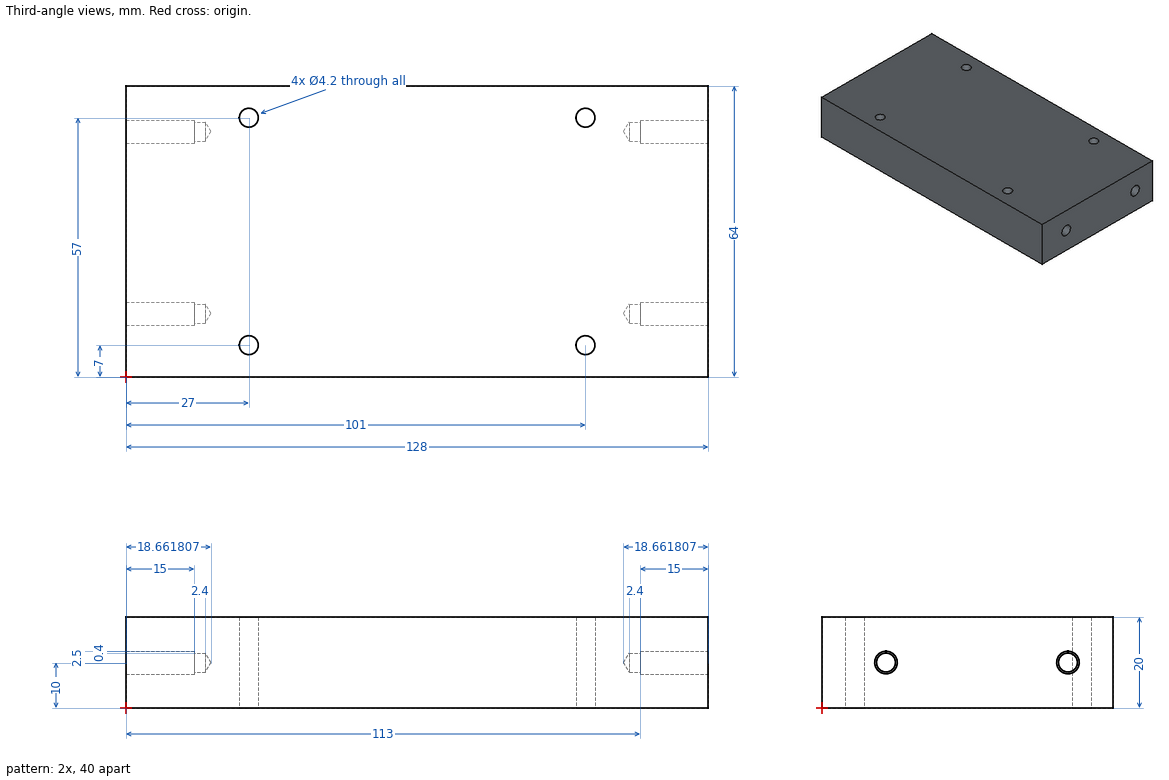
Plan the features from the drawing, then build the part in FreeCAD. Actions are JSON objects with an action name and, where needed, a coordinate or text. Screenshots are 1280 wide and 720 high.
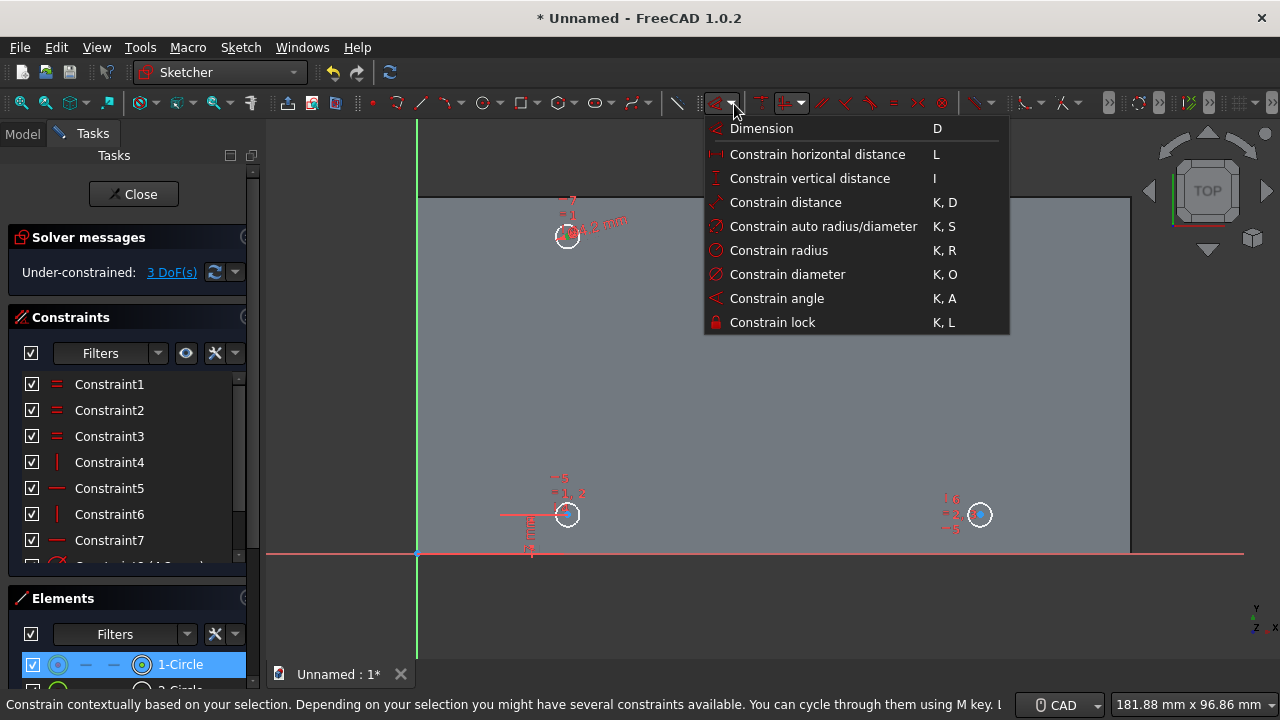
{"action": "left_click", "coordinate": [857, 154]}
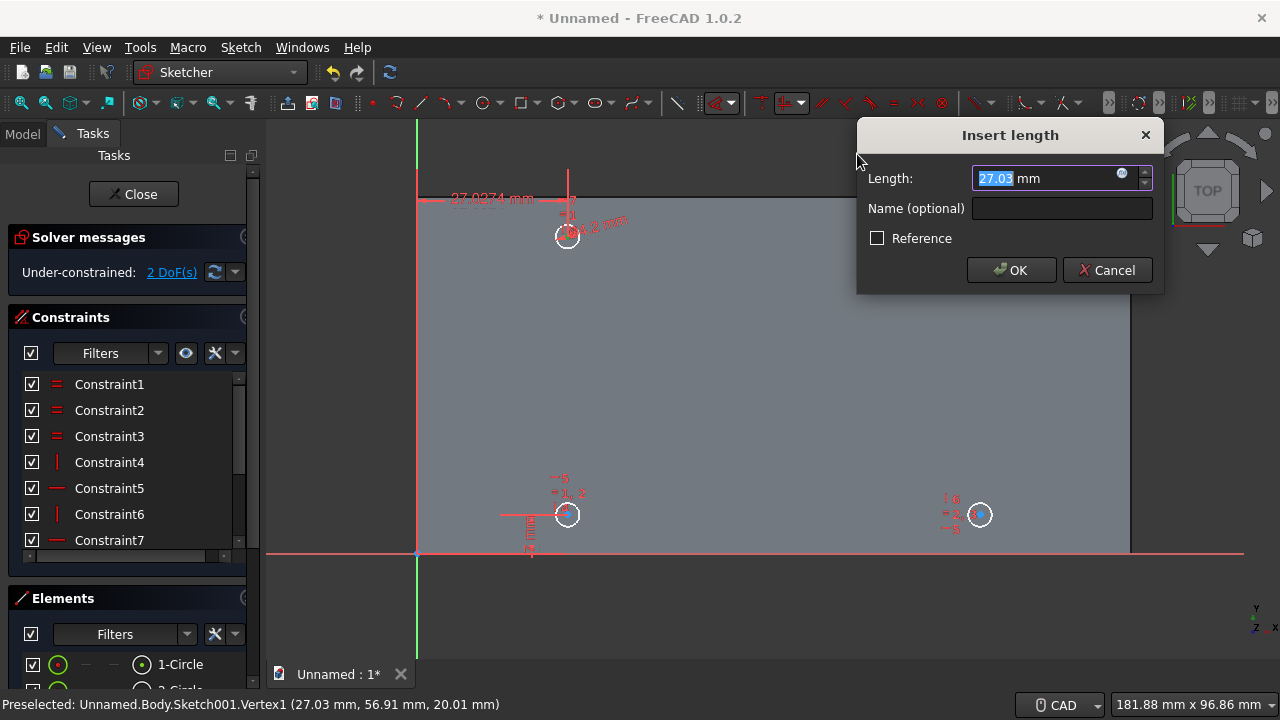
{"action": "type", "text": "27"}
{"action": "key", "text": "Return"}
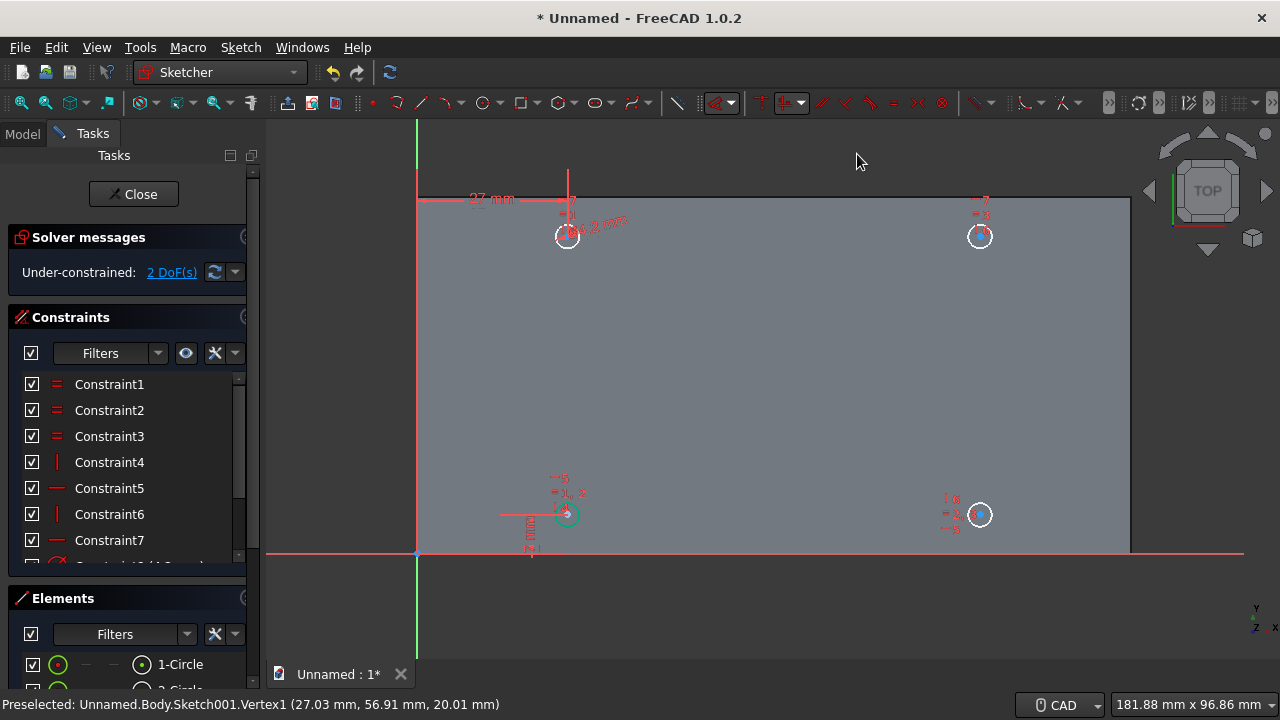
{"action": "left_click", "coordinate": [568, 237]}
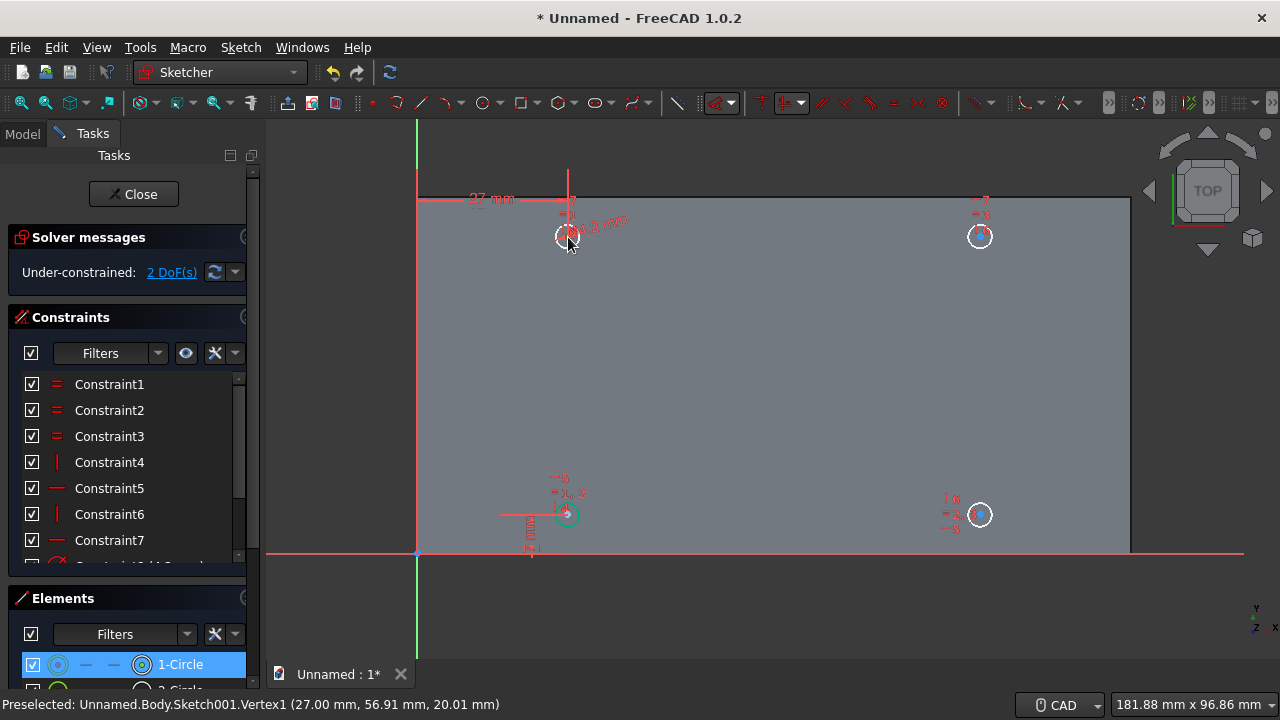
{"action": "left_click", "coordinate": [734, 104]}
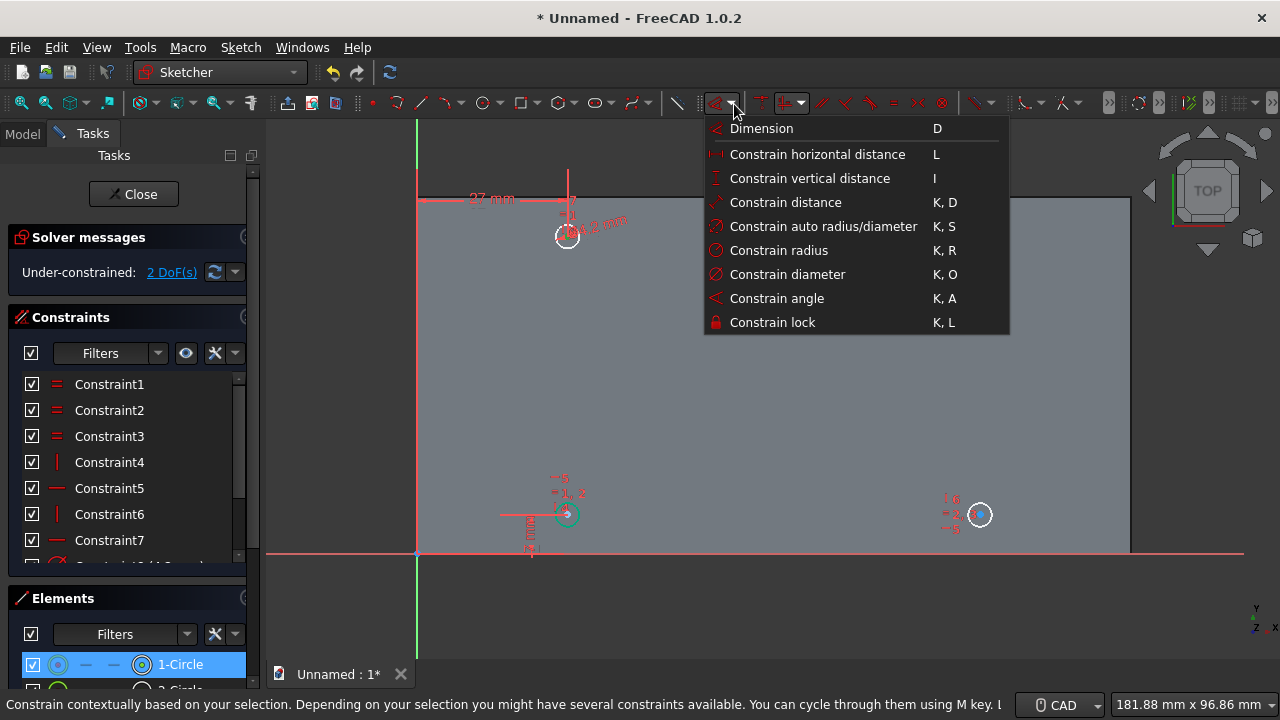
{"action": "left_click", "coordinate": [857, 178]}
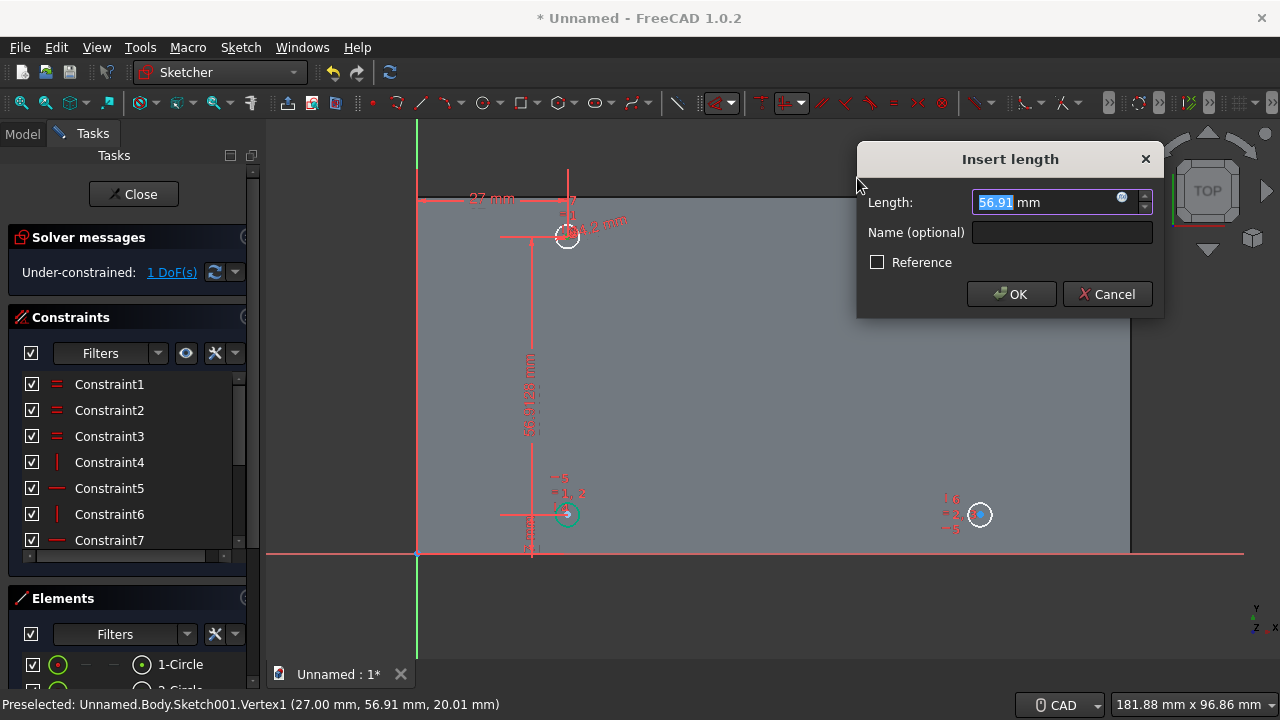
{"action": "type", "text": "57"}
{"action": "key", "text": "Return"}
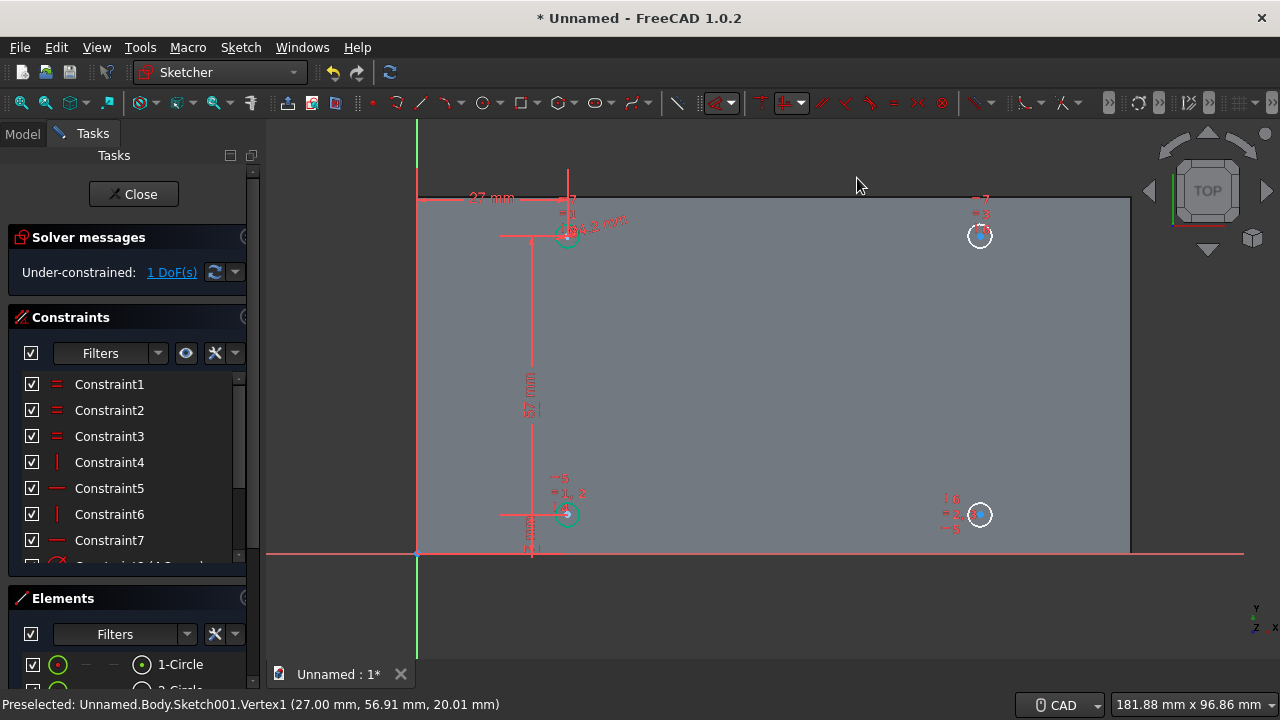
{"action": "left_click", "coordinate": [980, 515]}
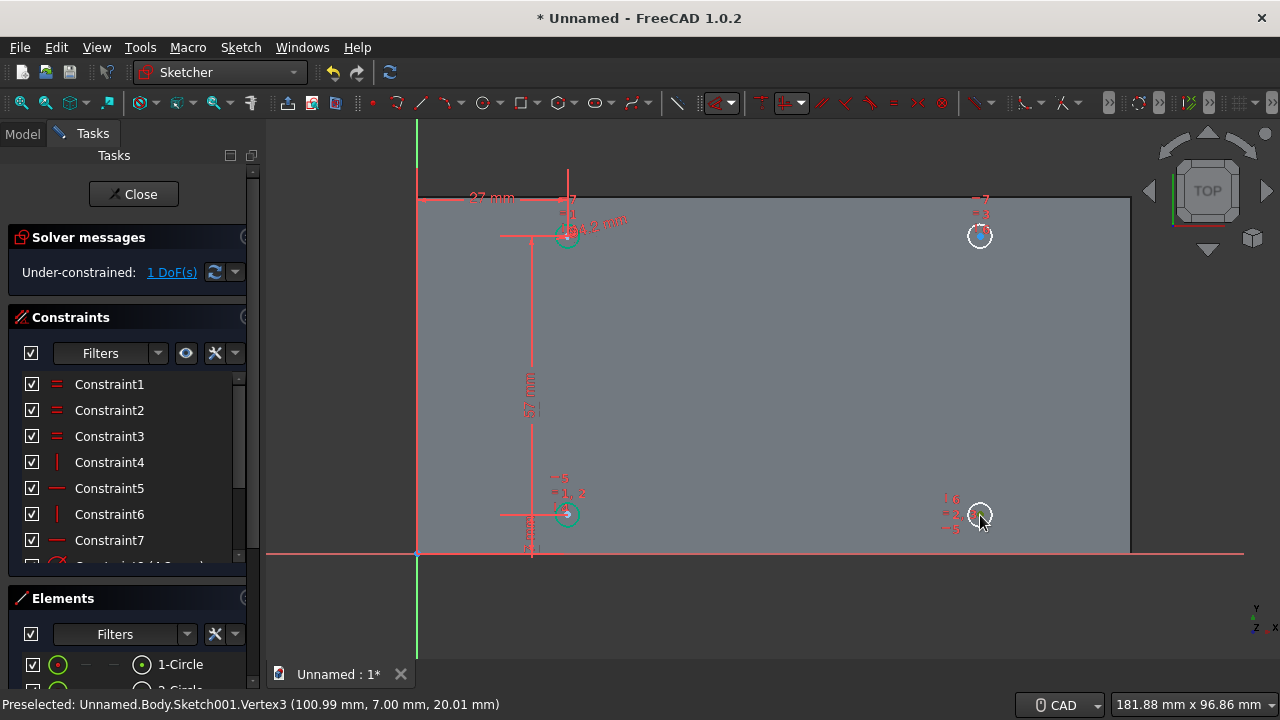
{"action": "left_click", "coordinate": [734, 104]}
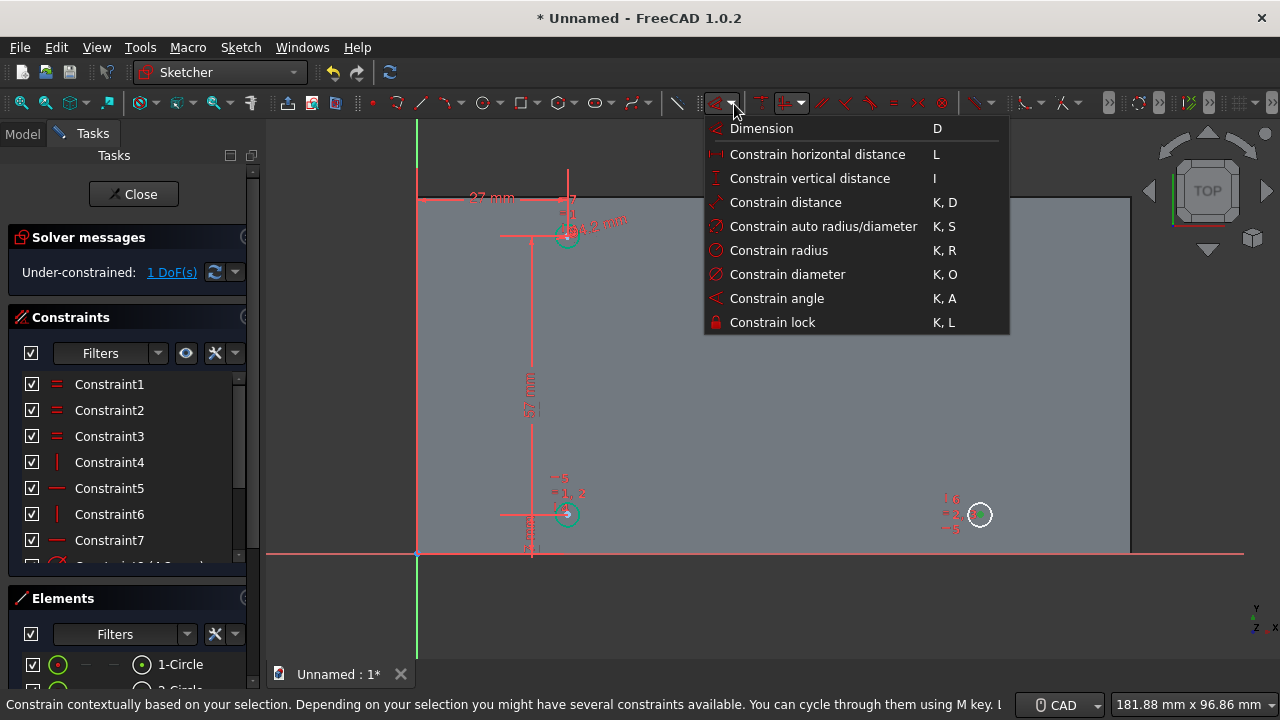
{"action": "left_click", "coordinate": [857, 154]}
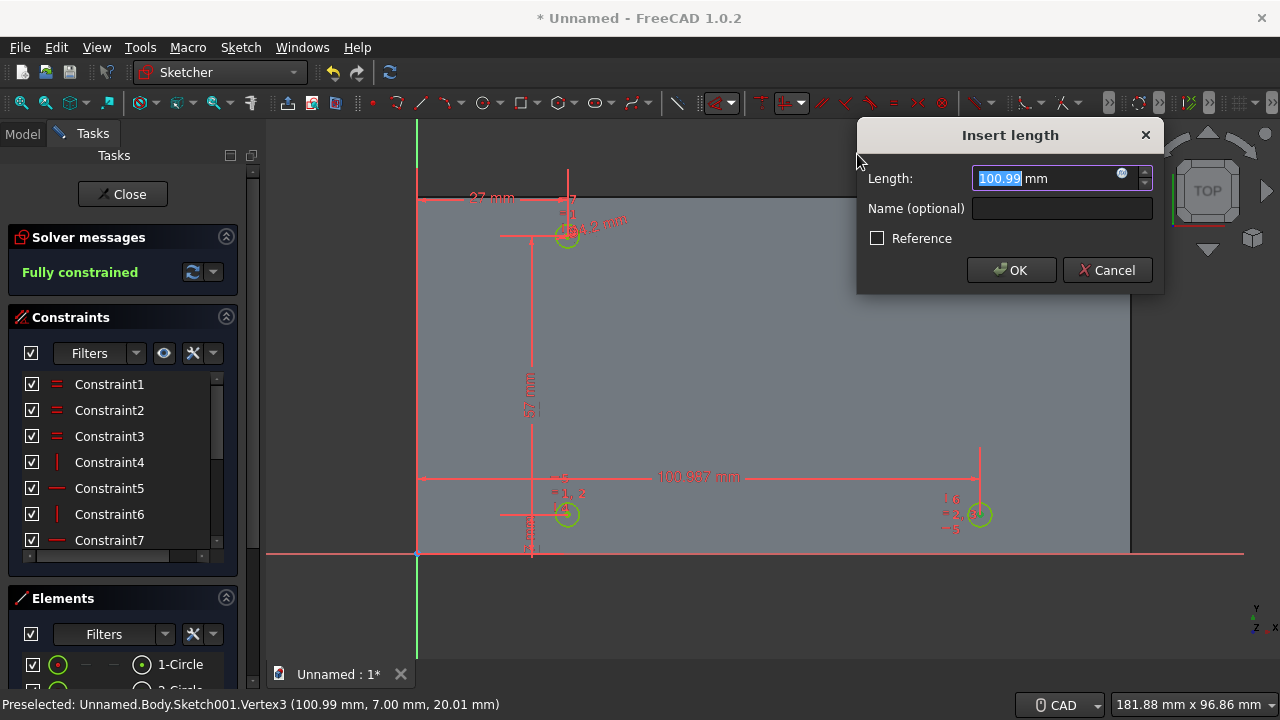
{"action": "type", "text": "101"}
{"action": "key", "text": "Return"}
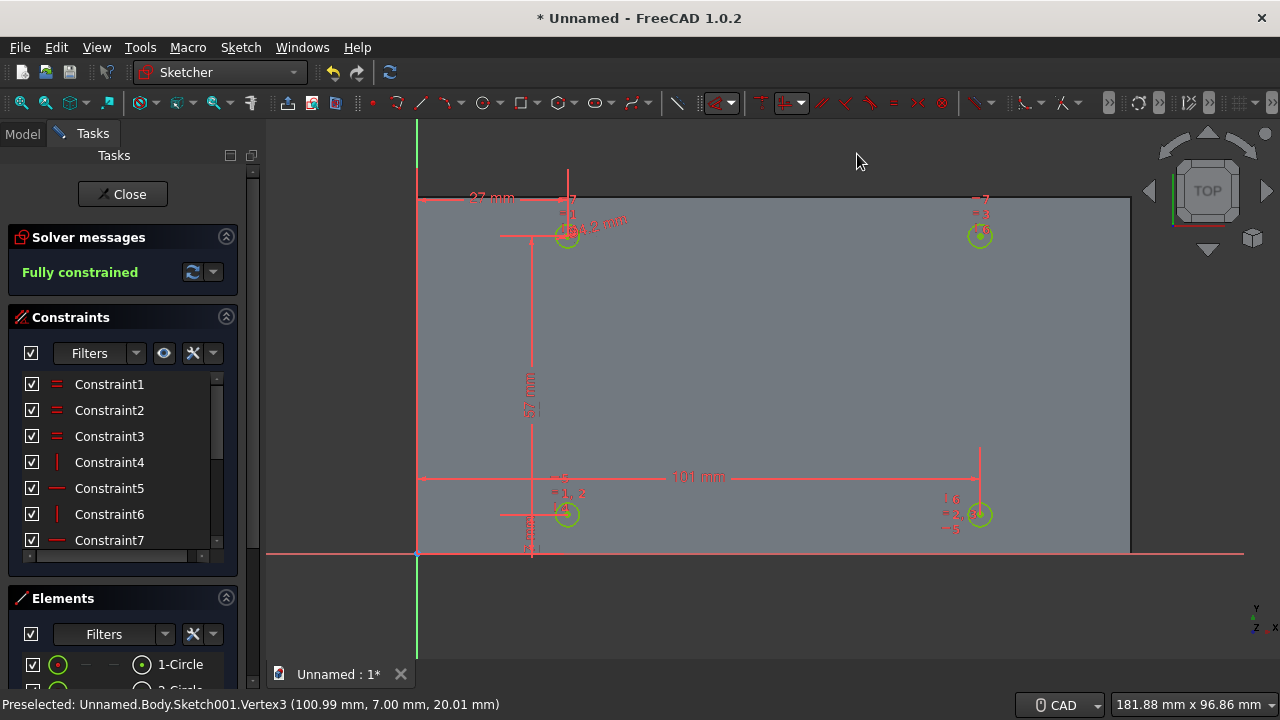
{"action": "left_click", "coordinate": [123, 194]}